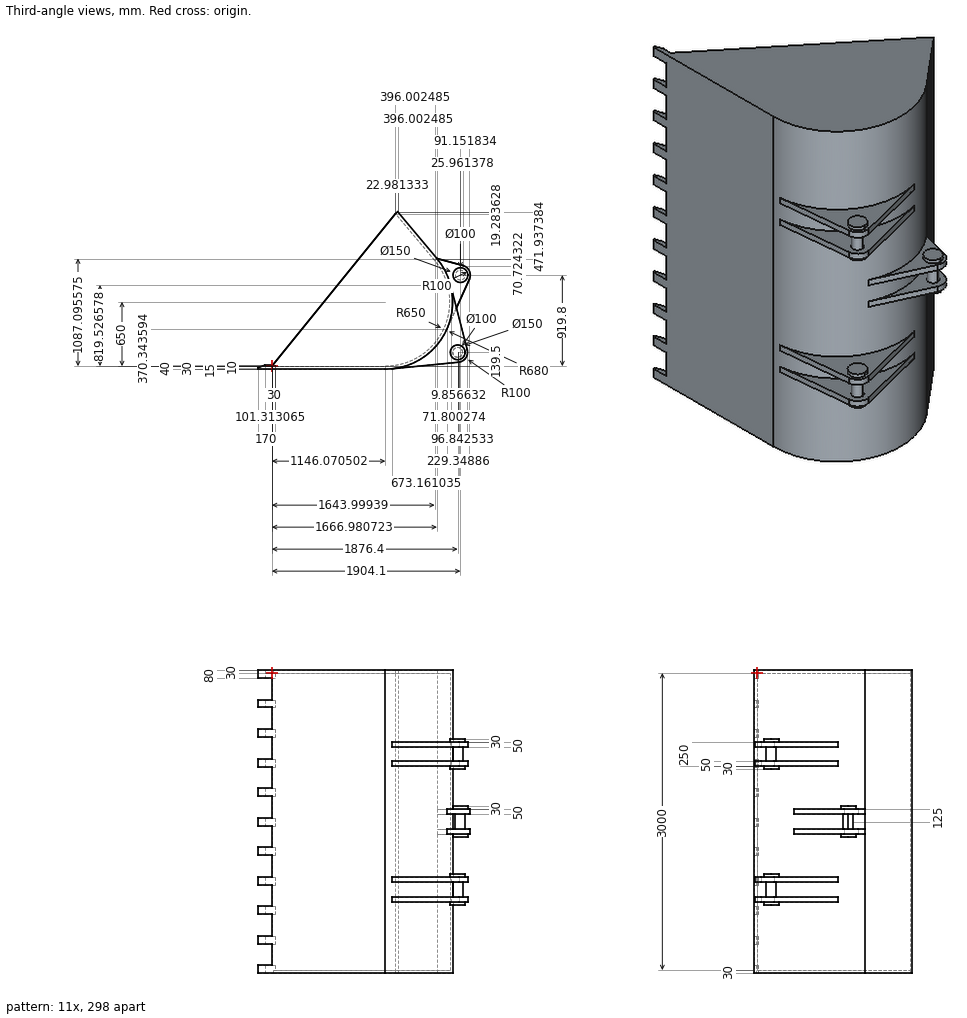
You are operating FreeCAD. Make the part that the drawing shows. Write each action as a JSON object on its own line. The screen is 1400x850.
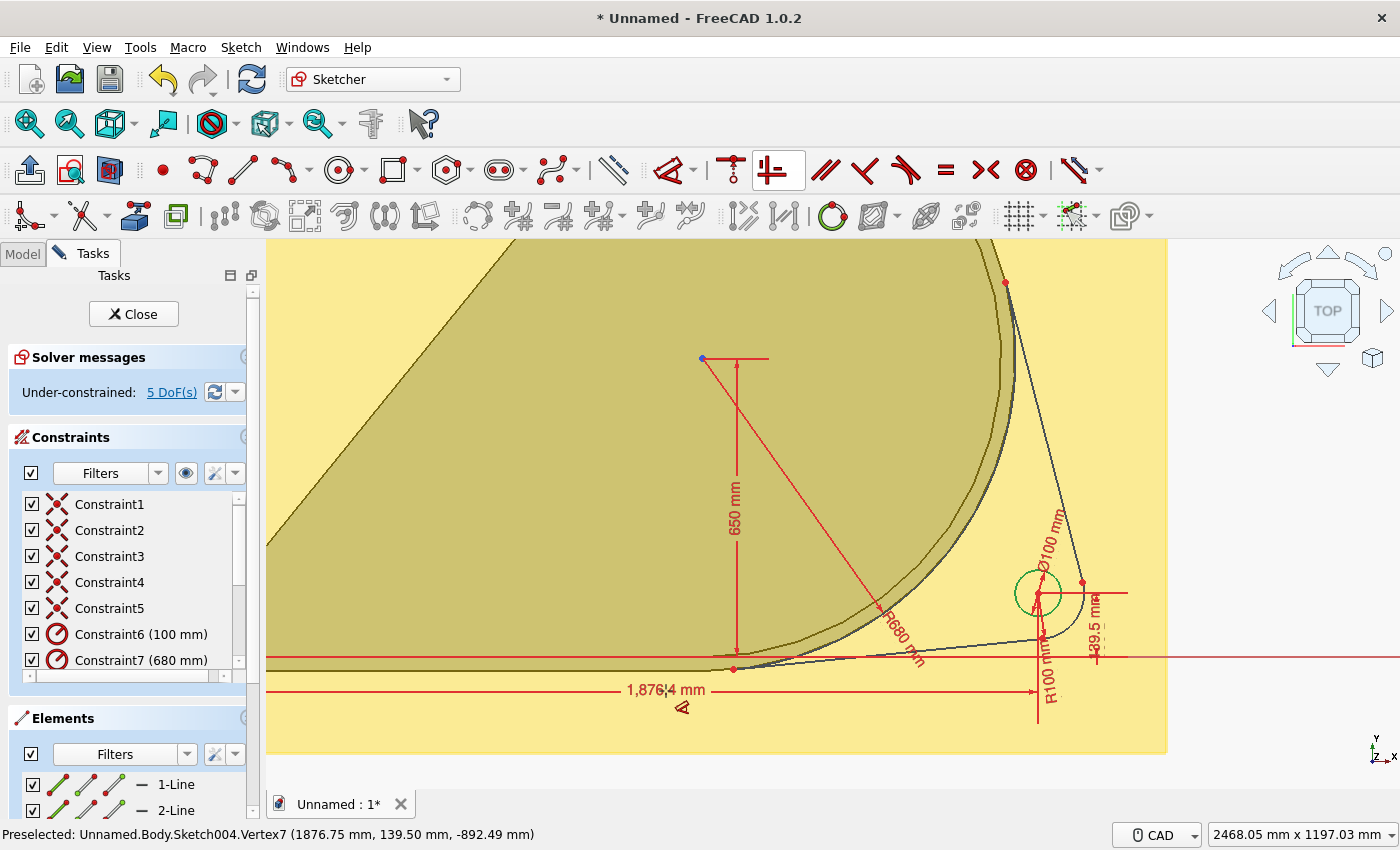
{"action": "scroll", "coordinate": [1043, 639], "scroll_direction": "up", "scroll_amount": 11}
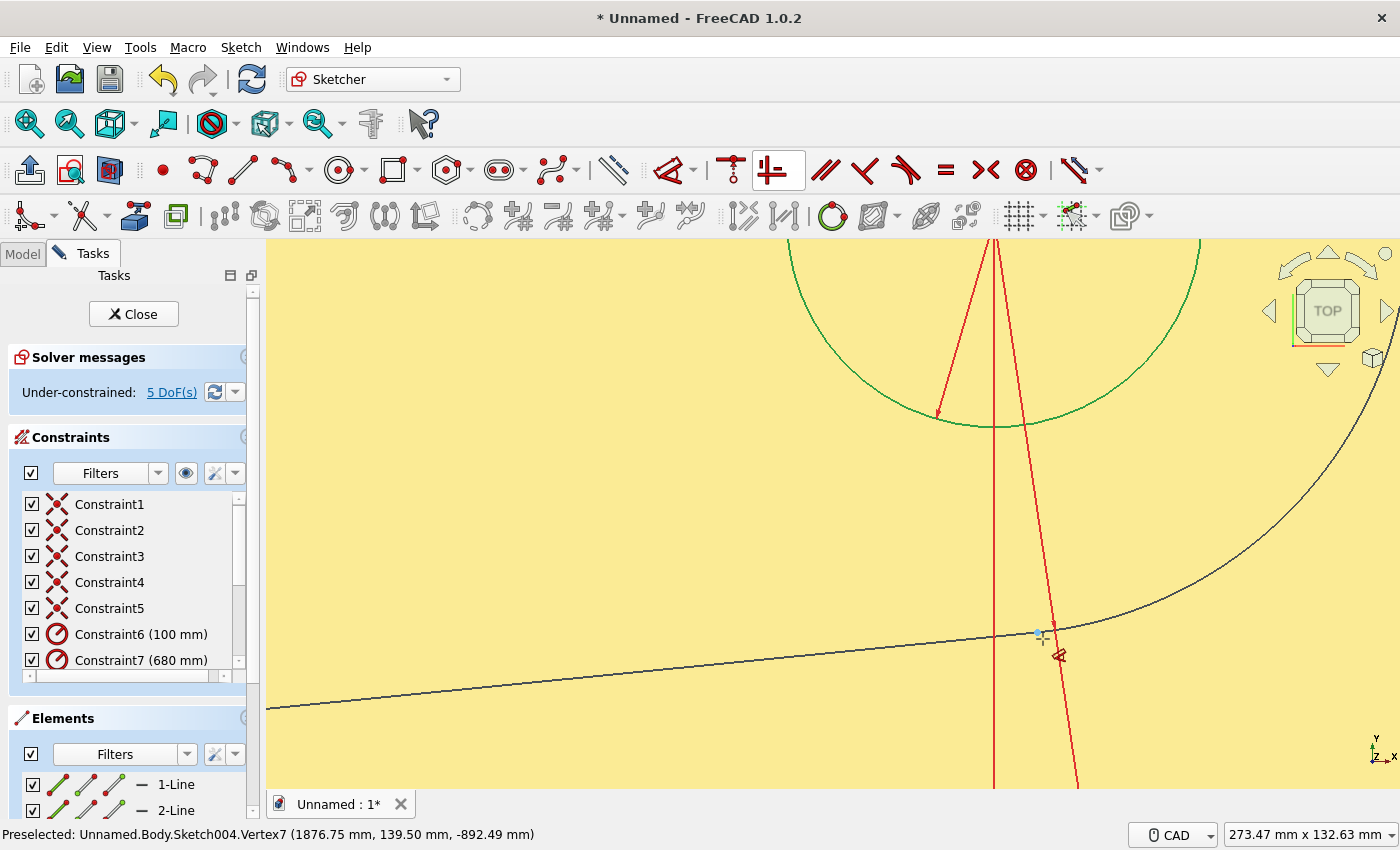
{"action": "left_click", "coordinate": [1037, 632]}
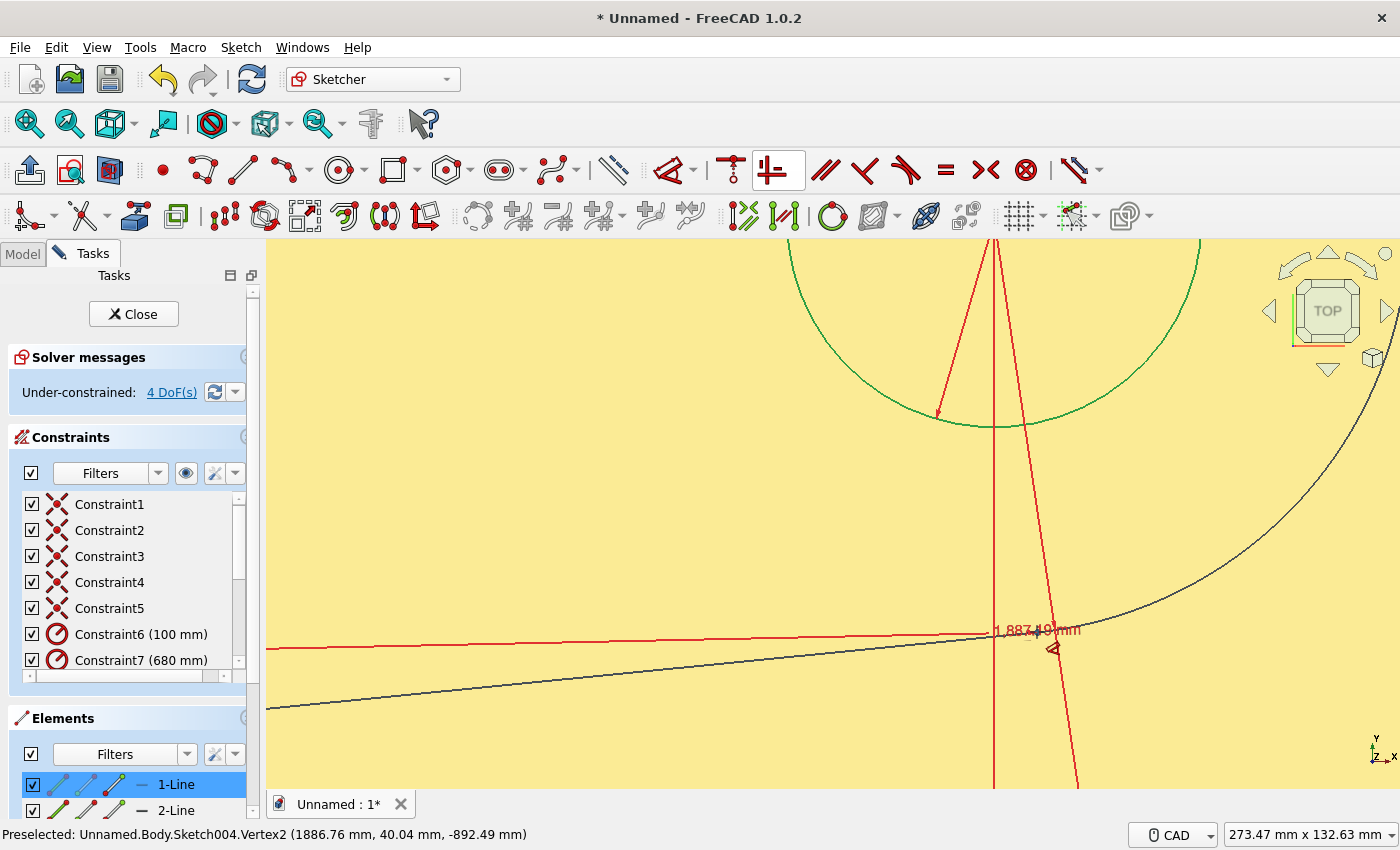
{"action": "scroll", "coordinate": [1042, 623], "scroll_direction": "down", "scroll_amount": 13}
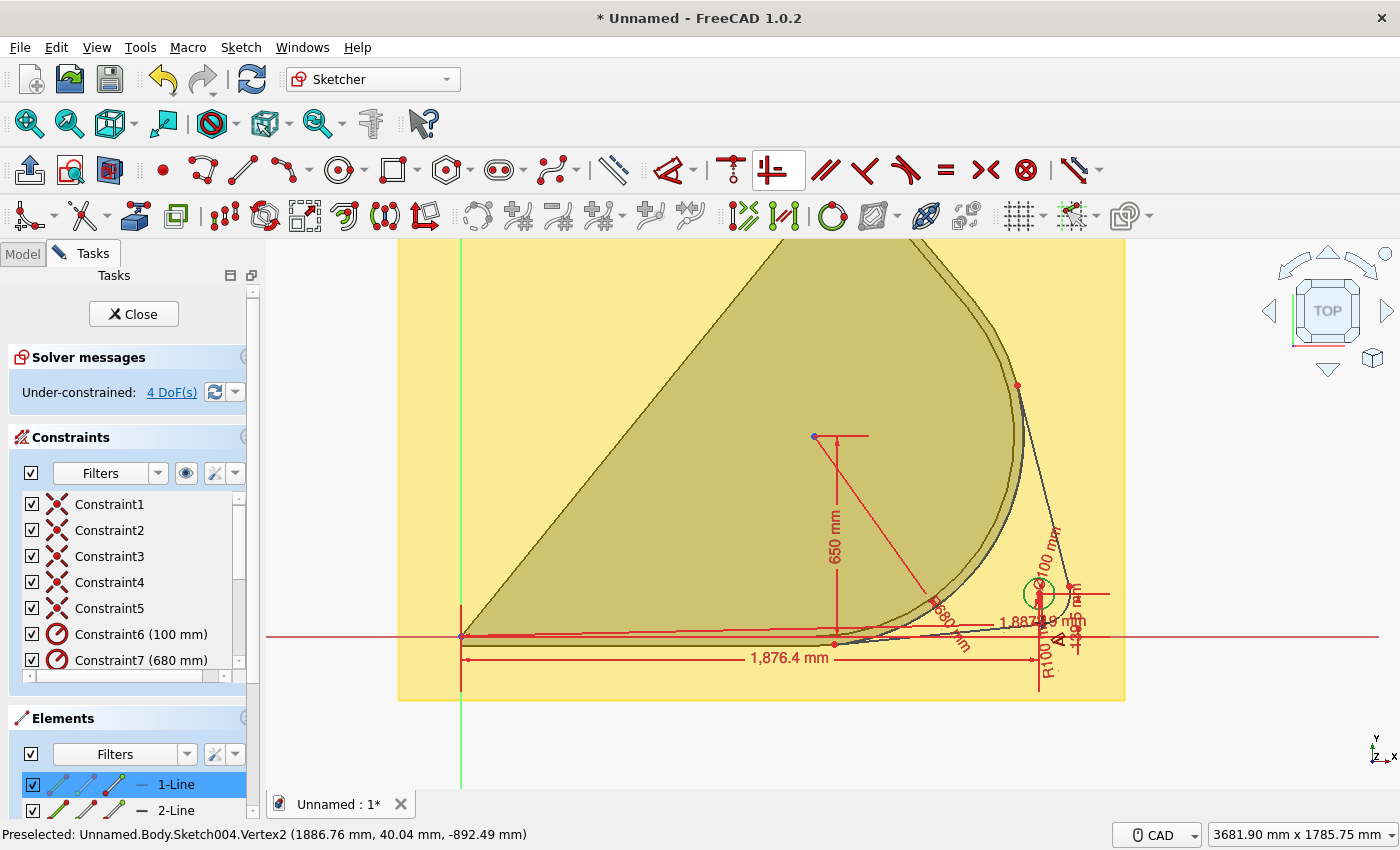
{"action": "scroll", "coordinate": [1039, 594], "scroll_direction": "up", "scroll_amount": 13}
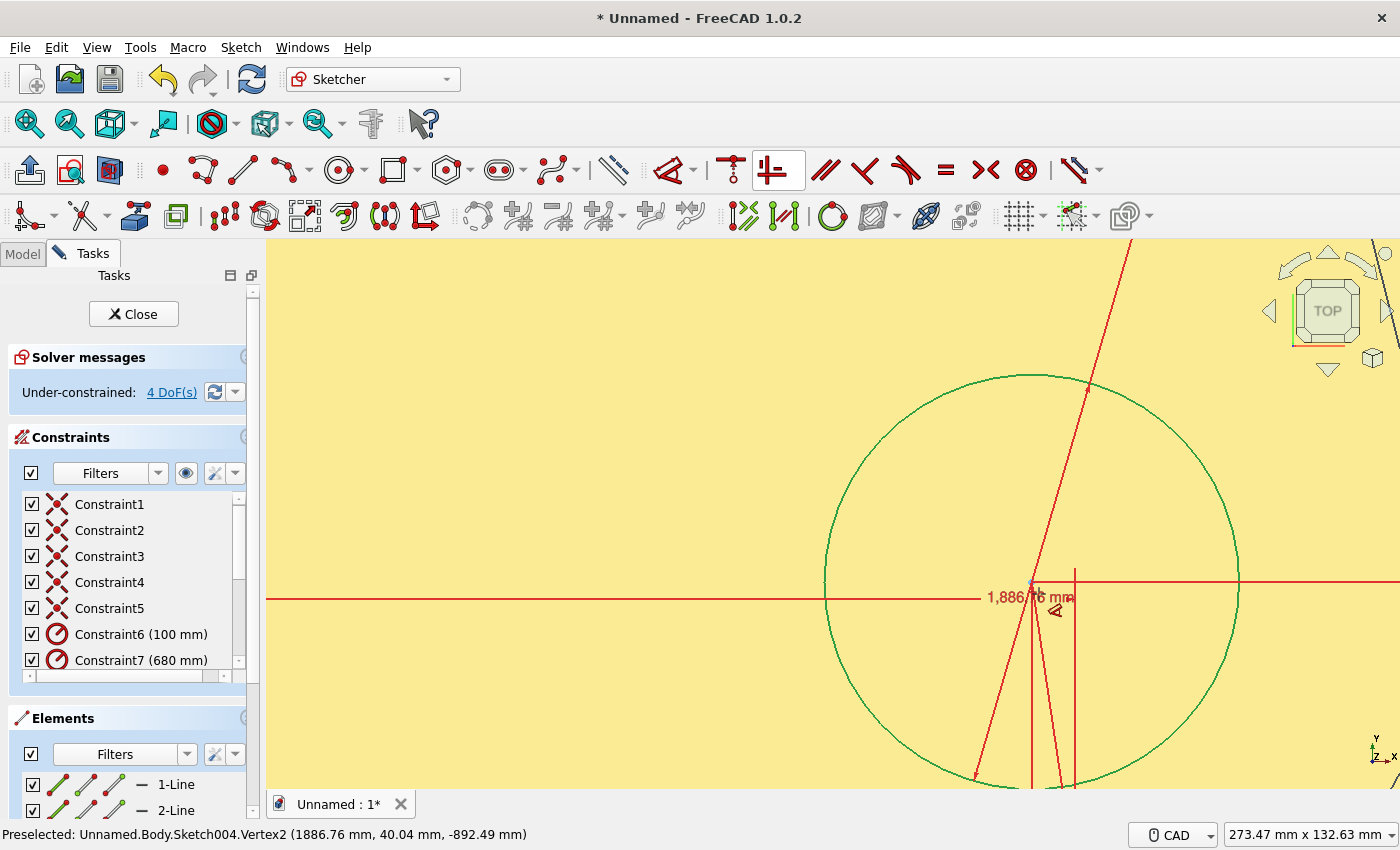
{"action": "left_click", "coordinate": [1032, 582]}
{"action": "left_click", "coordinate": [1053, 548]}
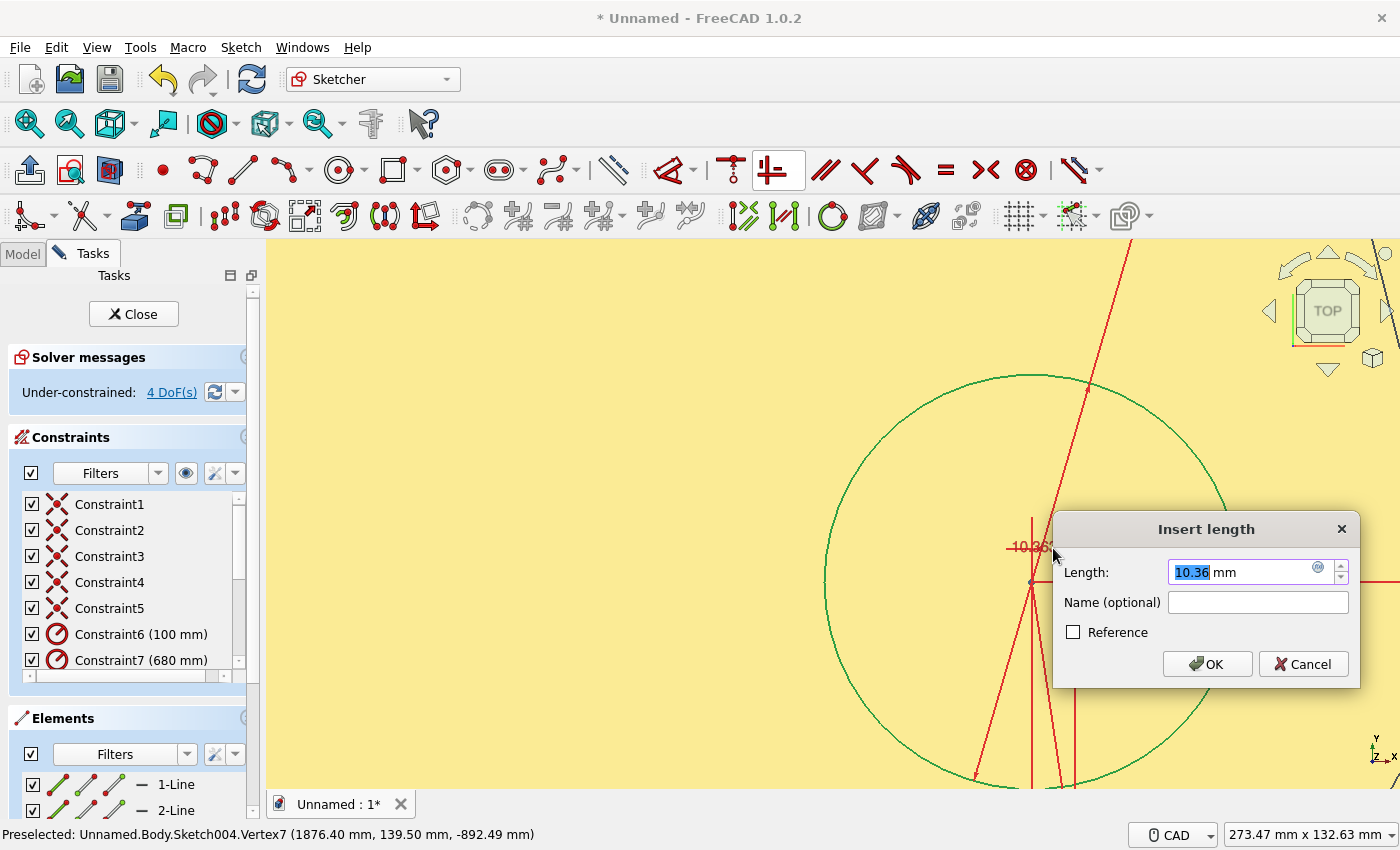
{"action": "type", "text": "9.856632"}
{"action": "key", "text": "Return"}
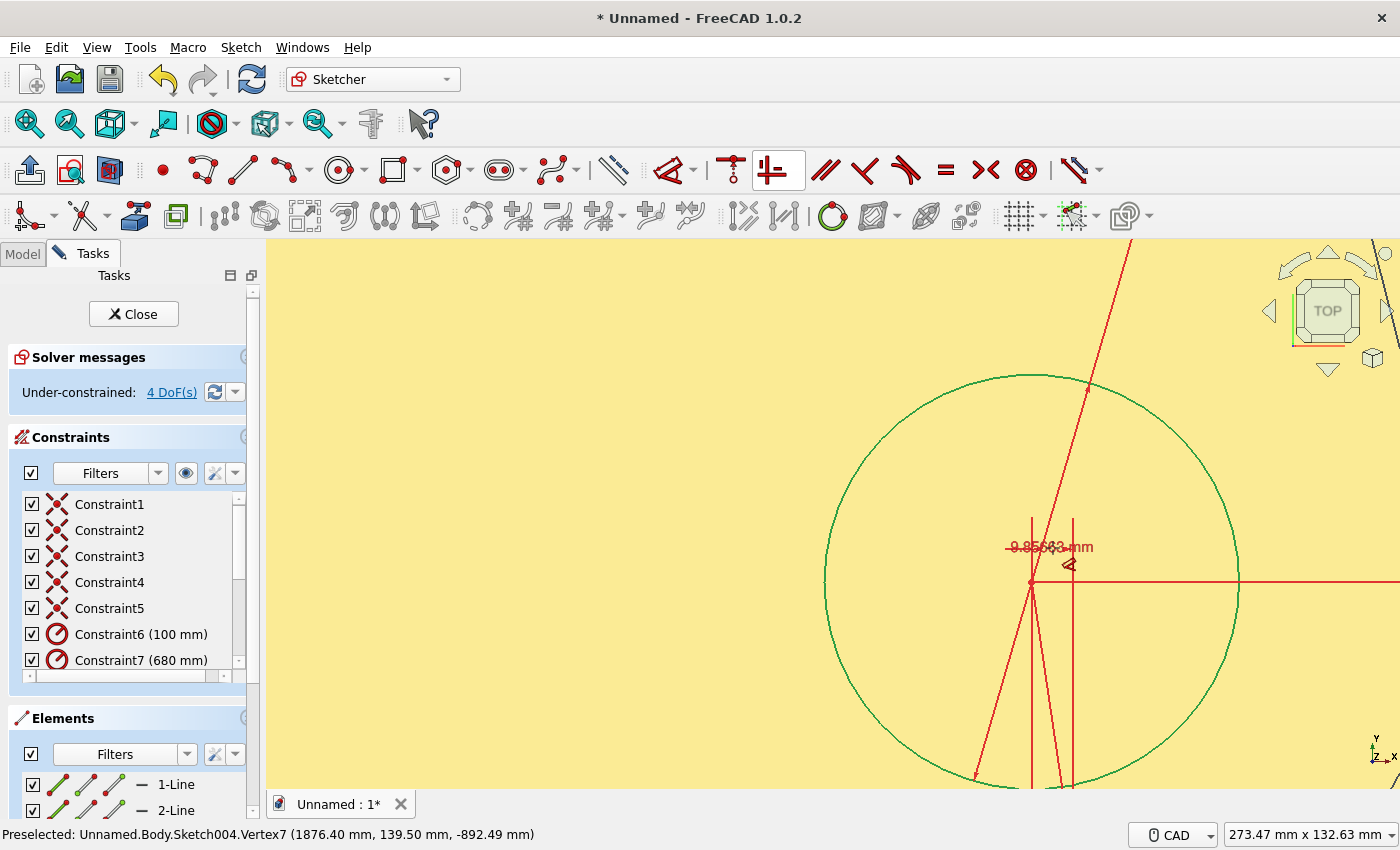
{"action": "scroll", "coordinate": [1039, 594], "scroll_direction": "down", "scroll_amount": 13}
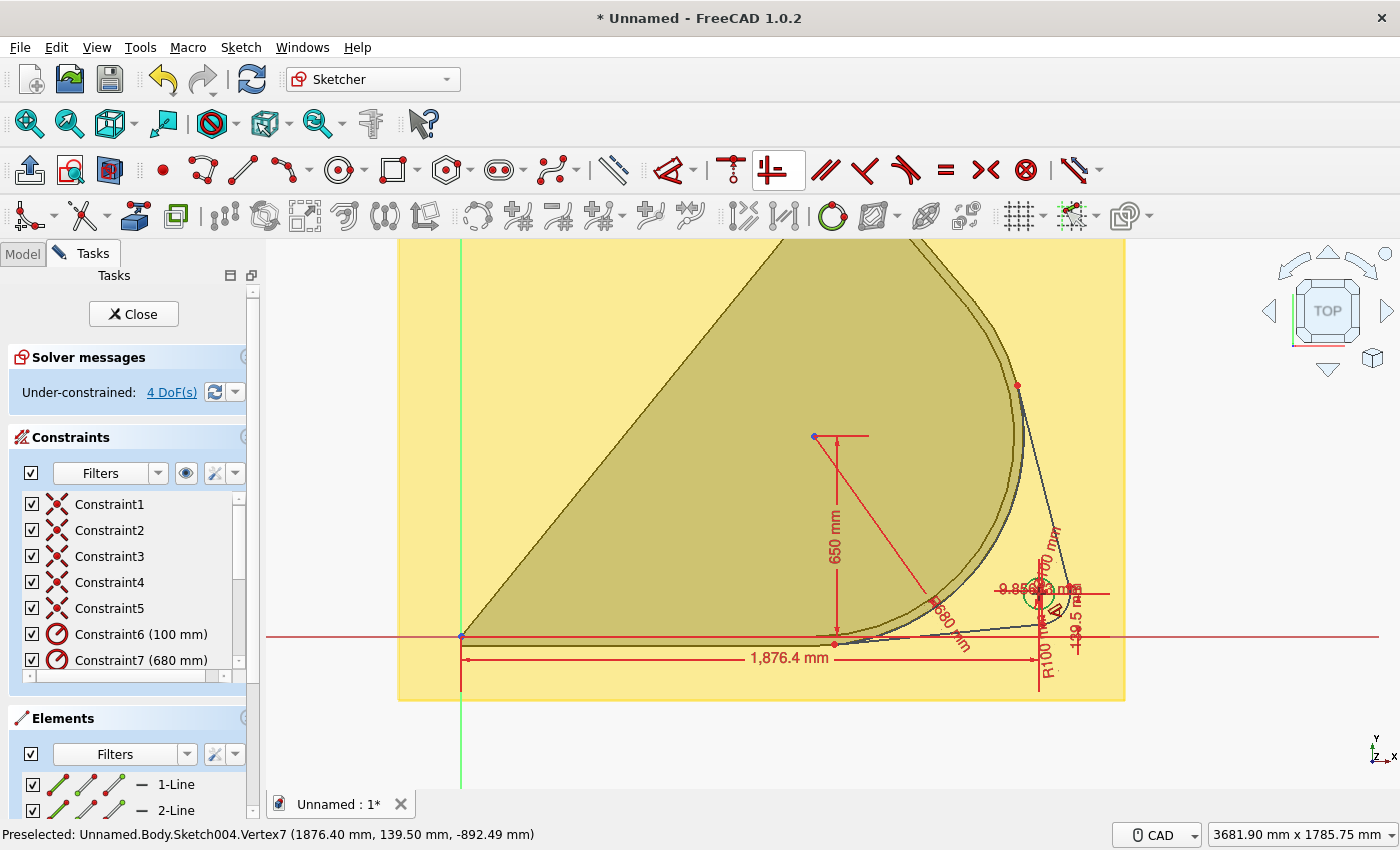
{"action": "scroll", "coordinate": [1069, 586], "scroll_direction": "up", "scroll_amount": 2}